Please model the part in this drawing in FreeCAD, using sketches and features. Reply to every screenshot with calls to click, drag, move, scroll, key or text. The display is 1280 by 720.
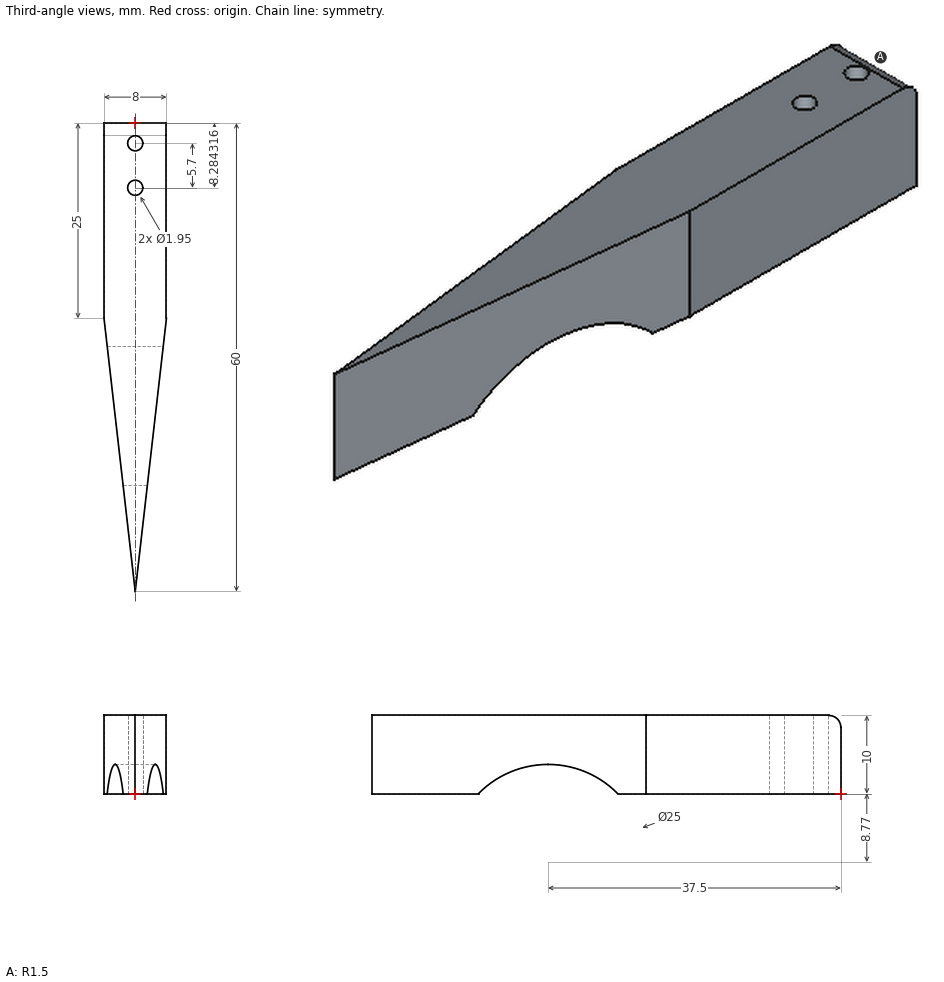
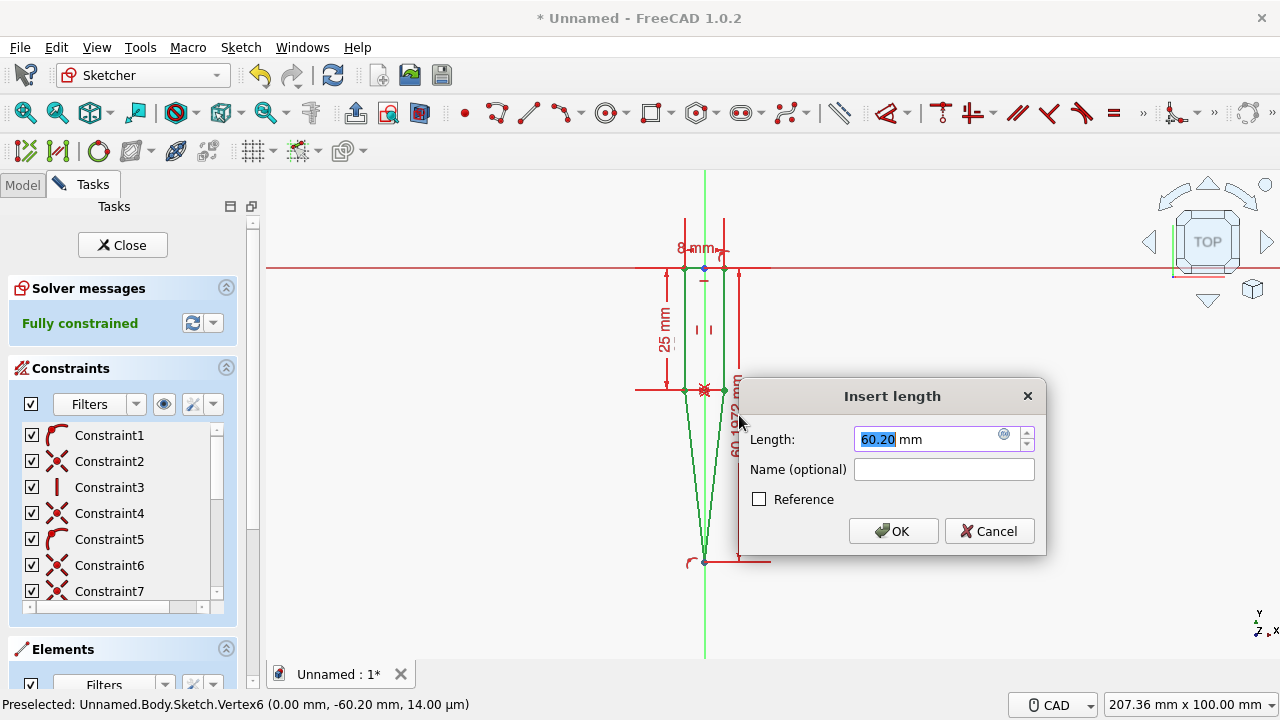
text(60)
key(Return)
key(Escape)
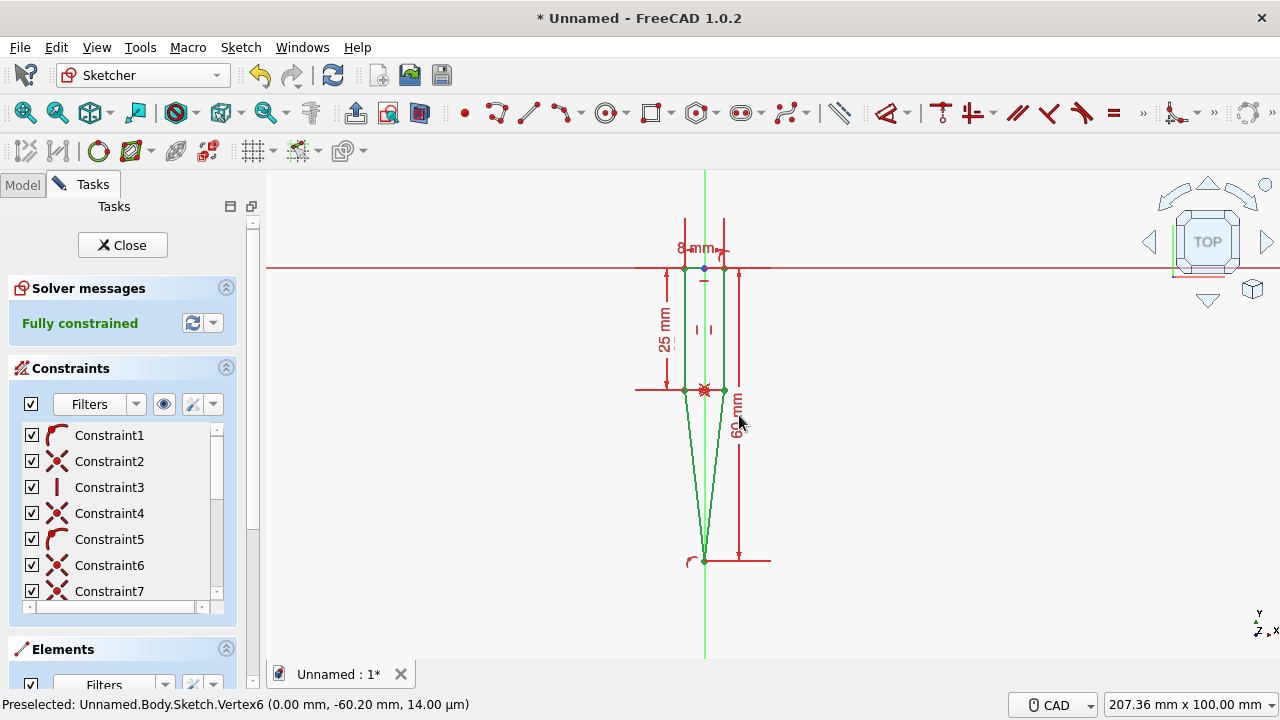
click(123, 245)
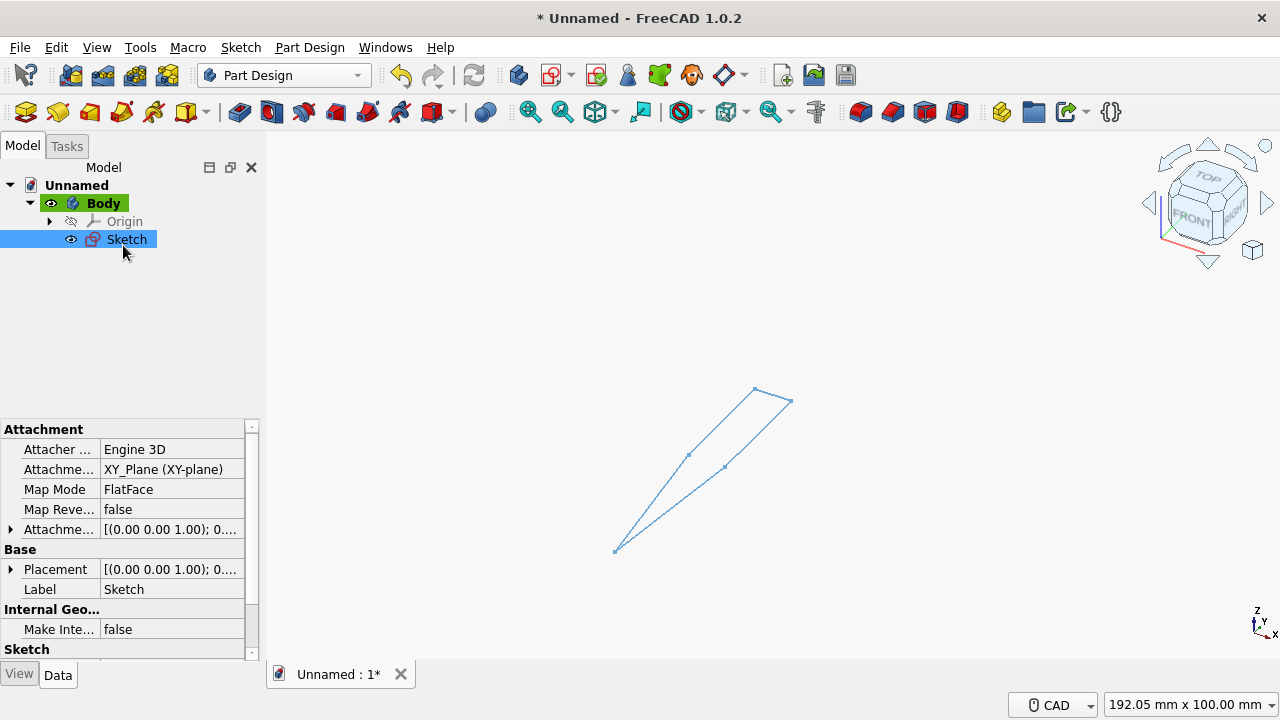
click(26, 112)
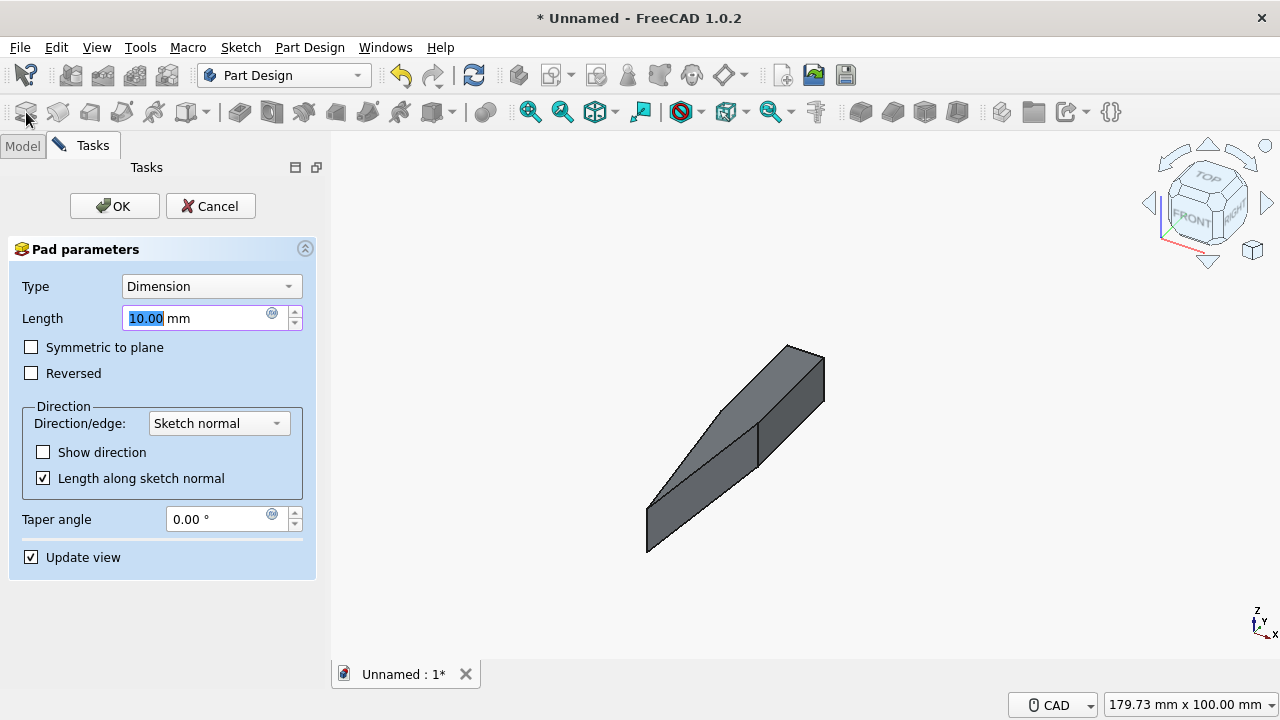
text(10)
key(Tab)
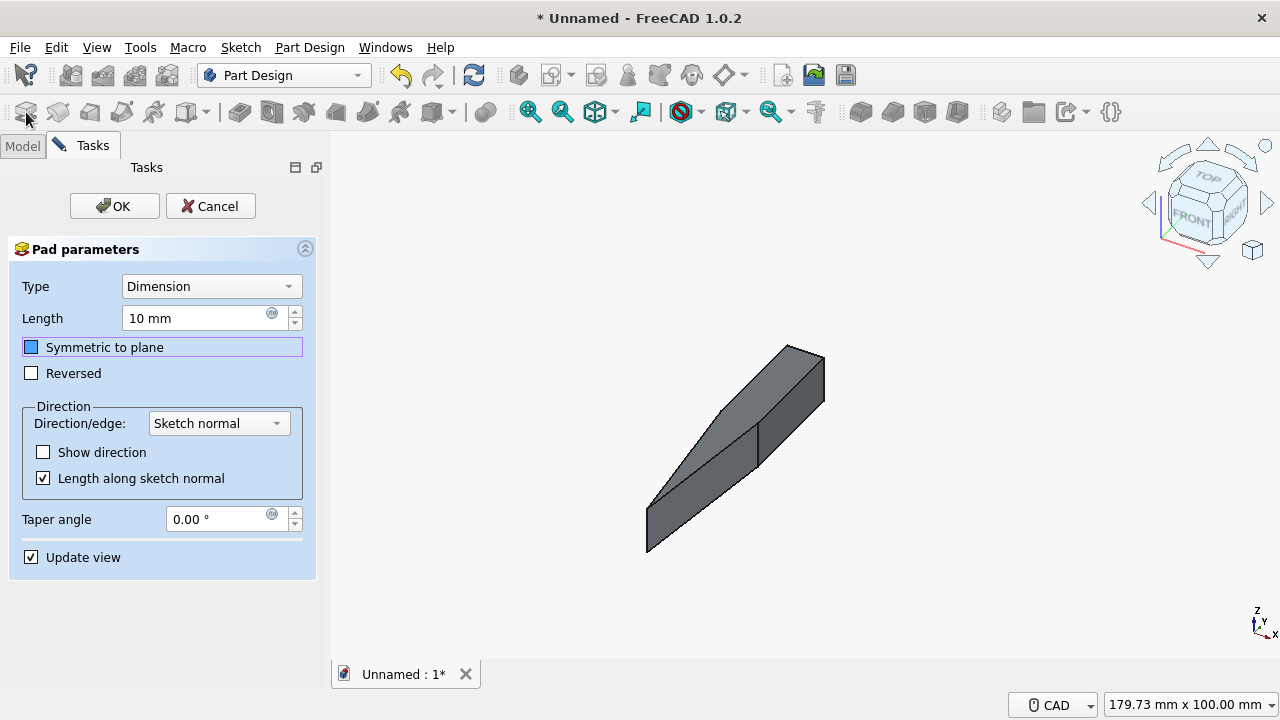
click(115, 206)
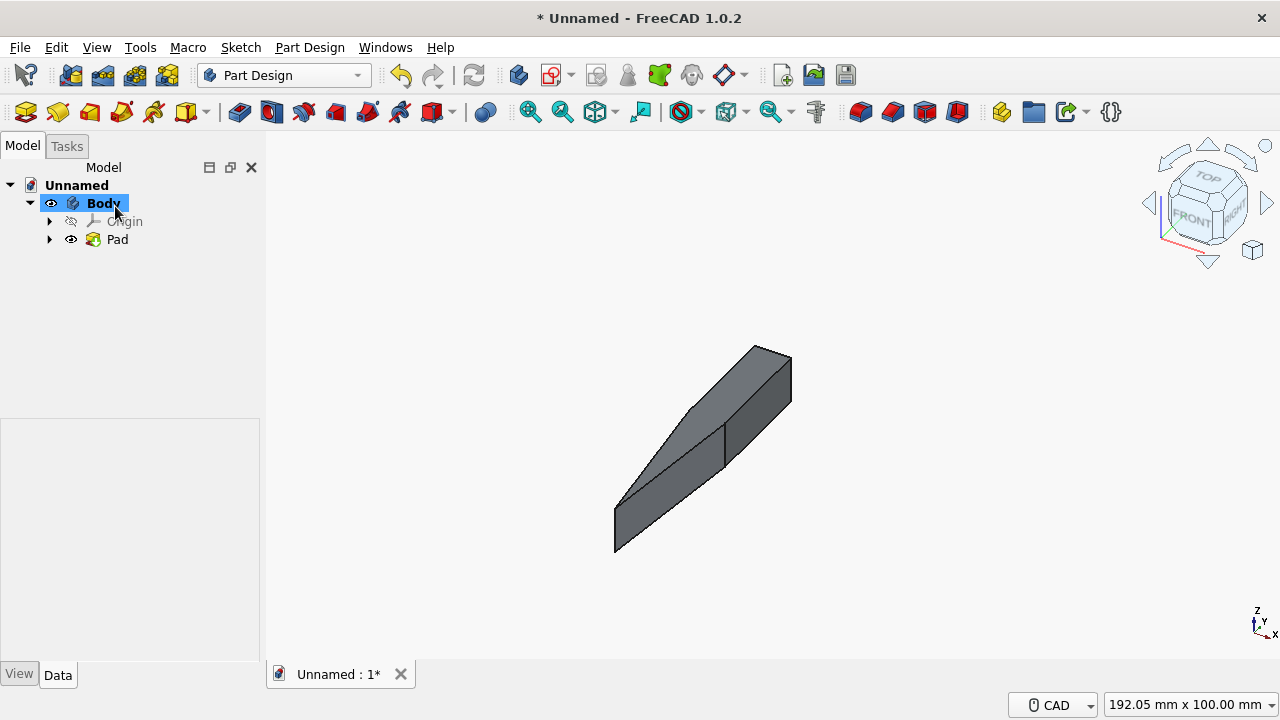
key(v)
key(f)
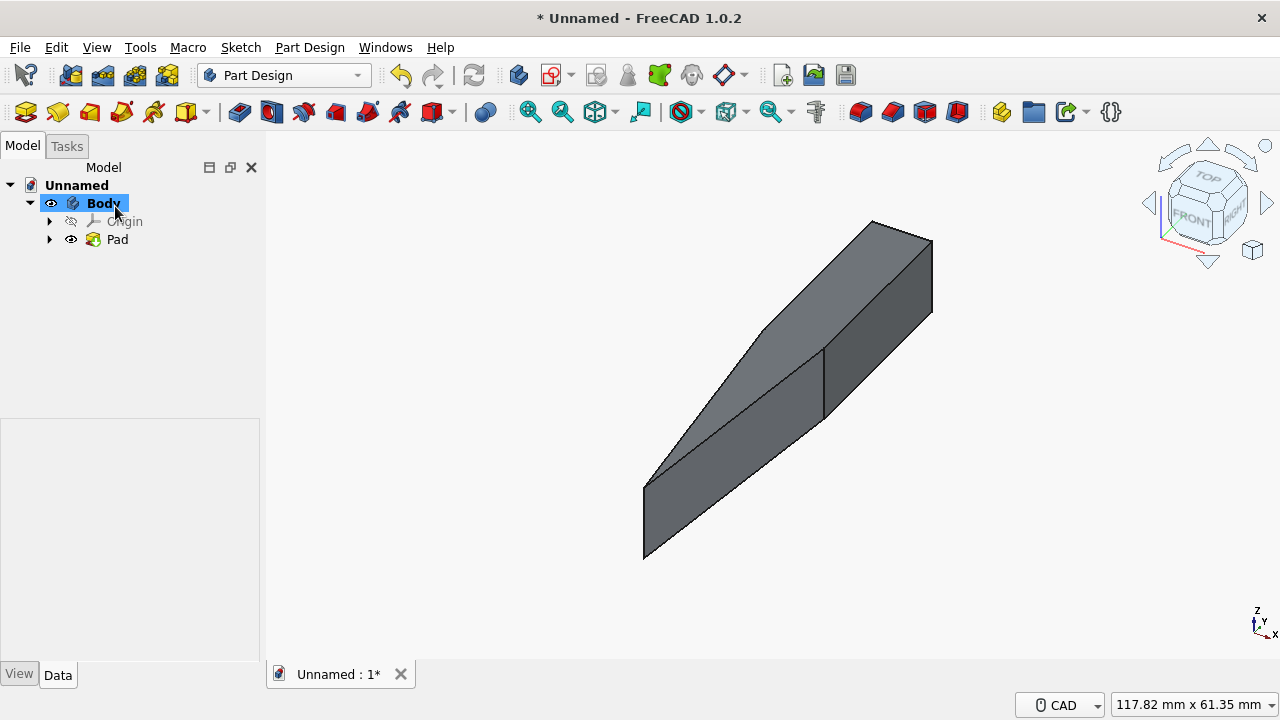
click(884, 249)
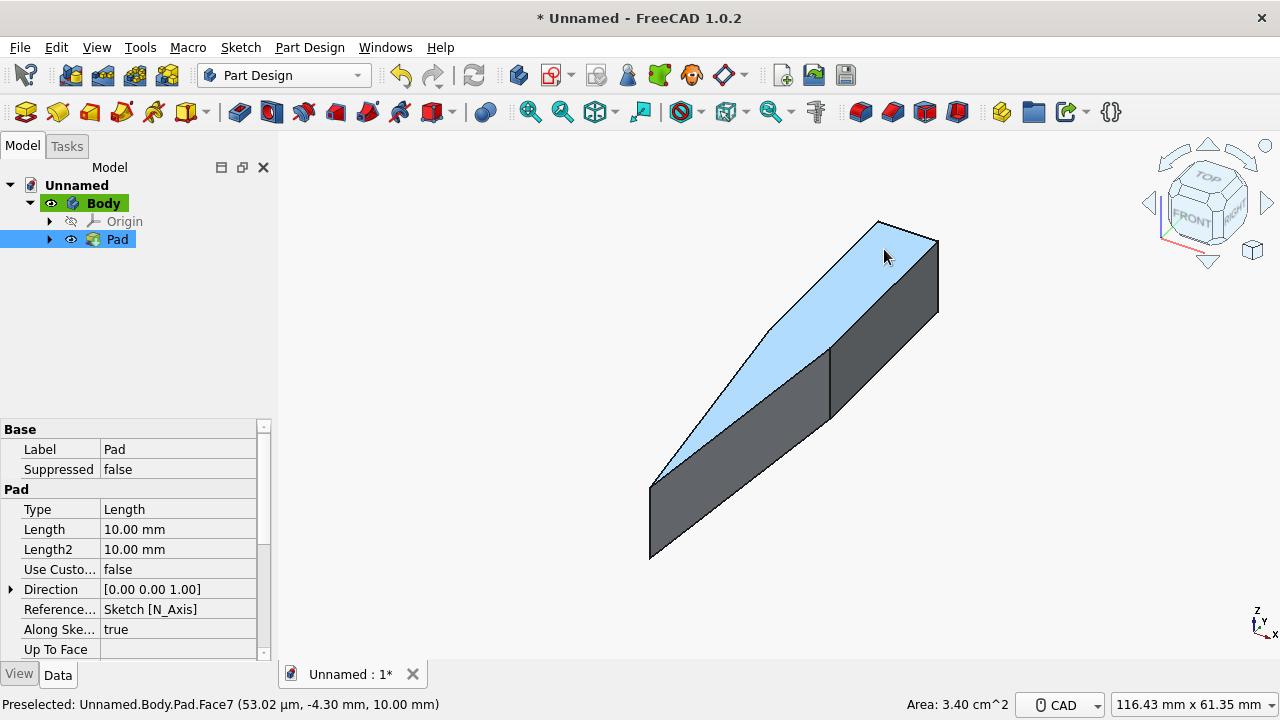
click(552, 76)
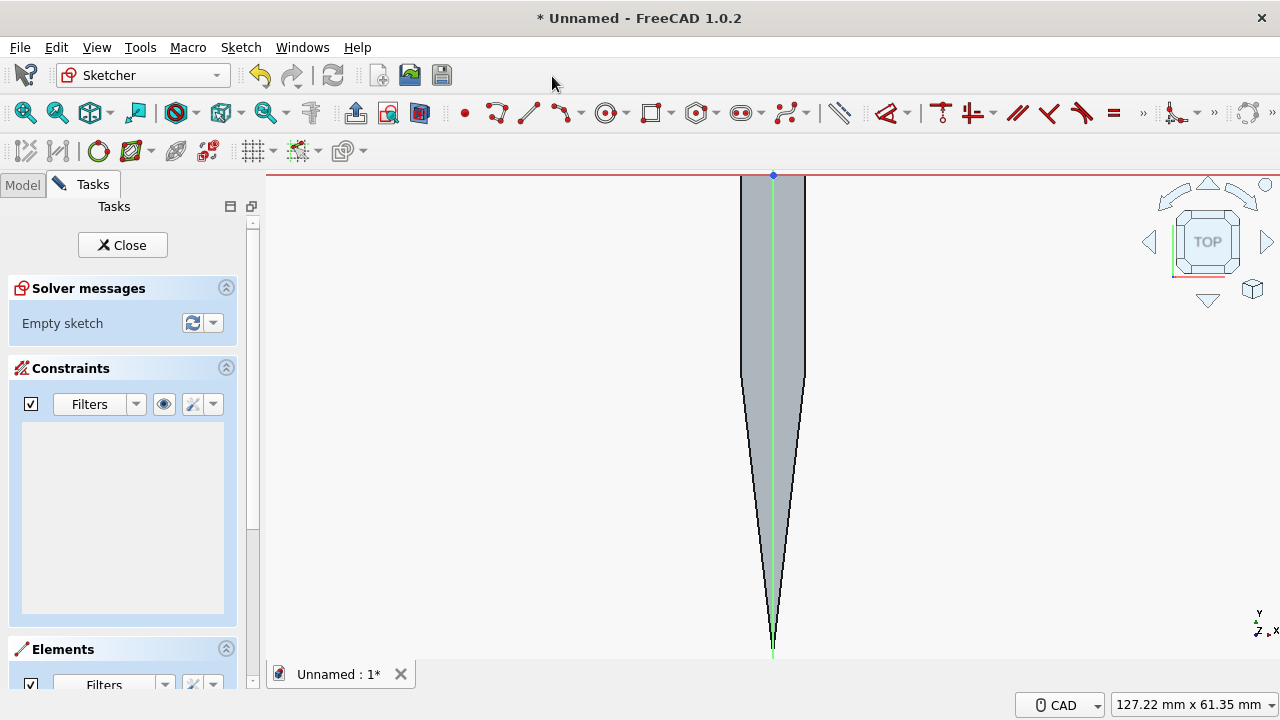
scroll(704, 414, down, 5)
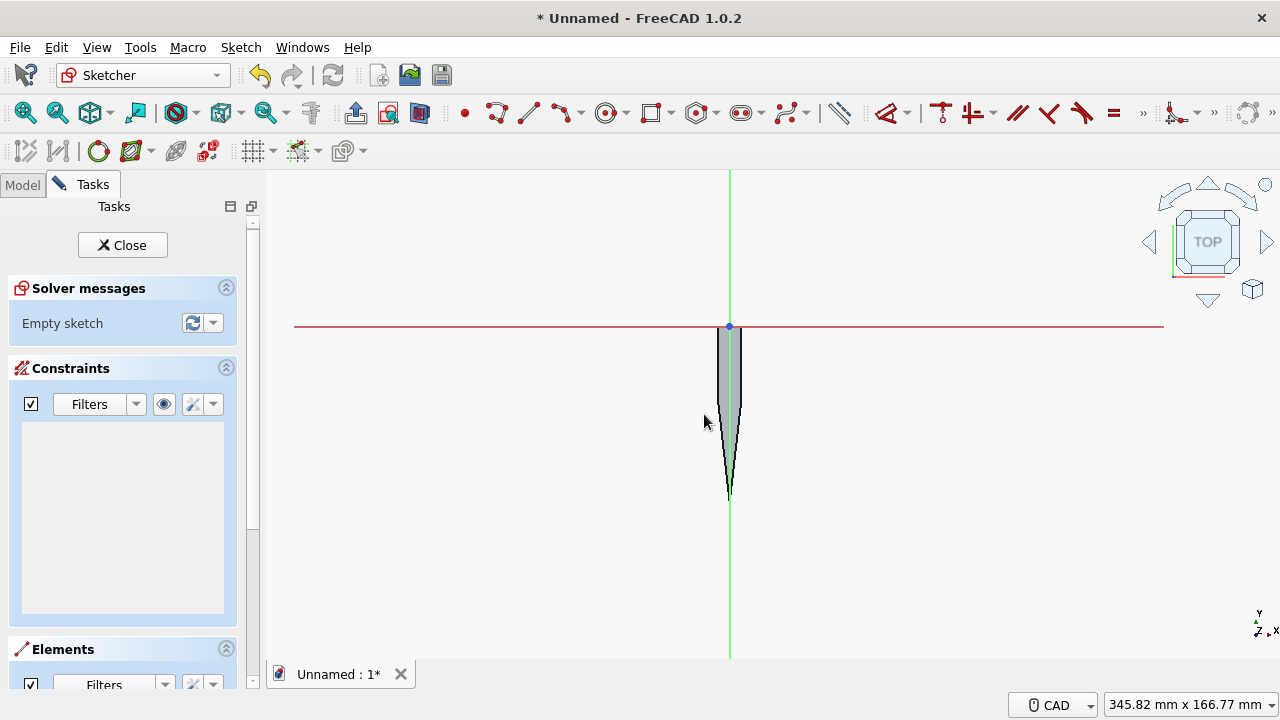
scroll(732, 333, up, 12)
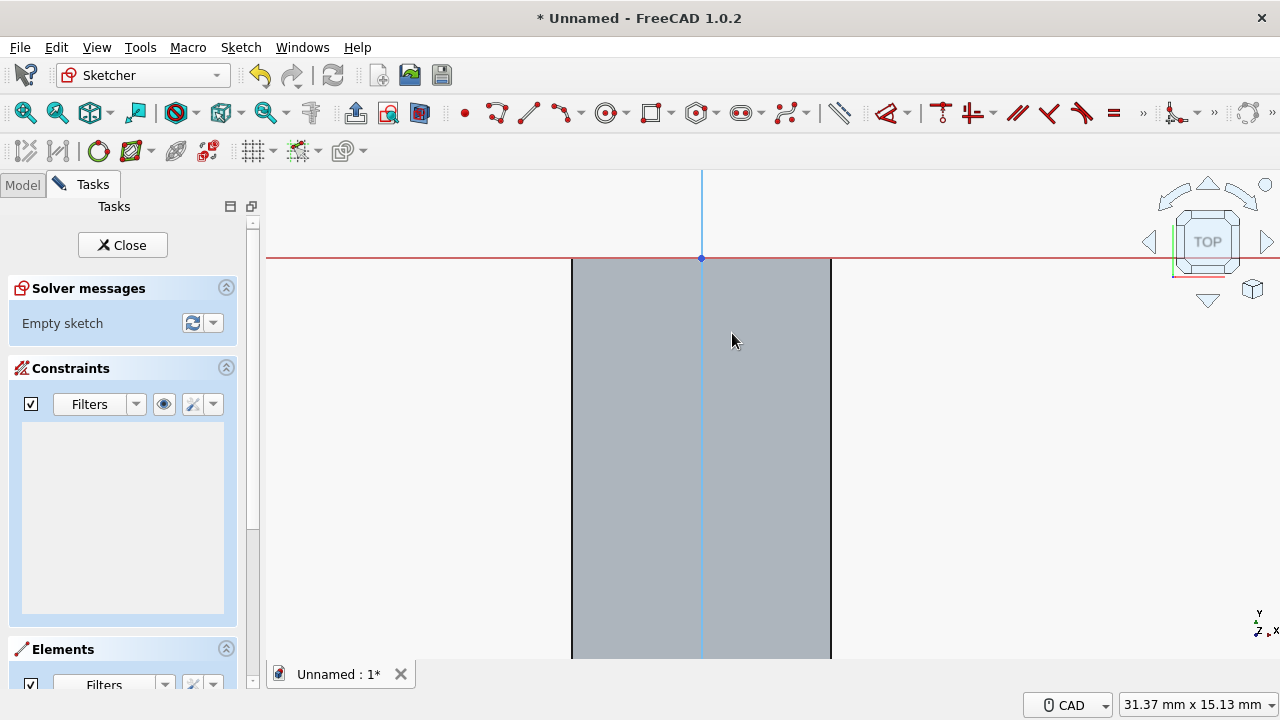
key(g)
key(c)